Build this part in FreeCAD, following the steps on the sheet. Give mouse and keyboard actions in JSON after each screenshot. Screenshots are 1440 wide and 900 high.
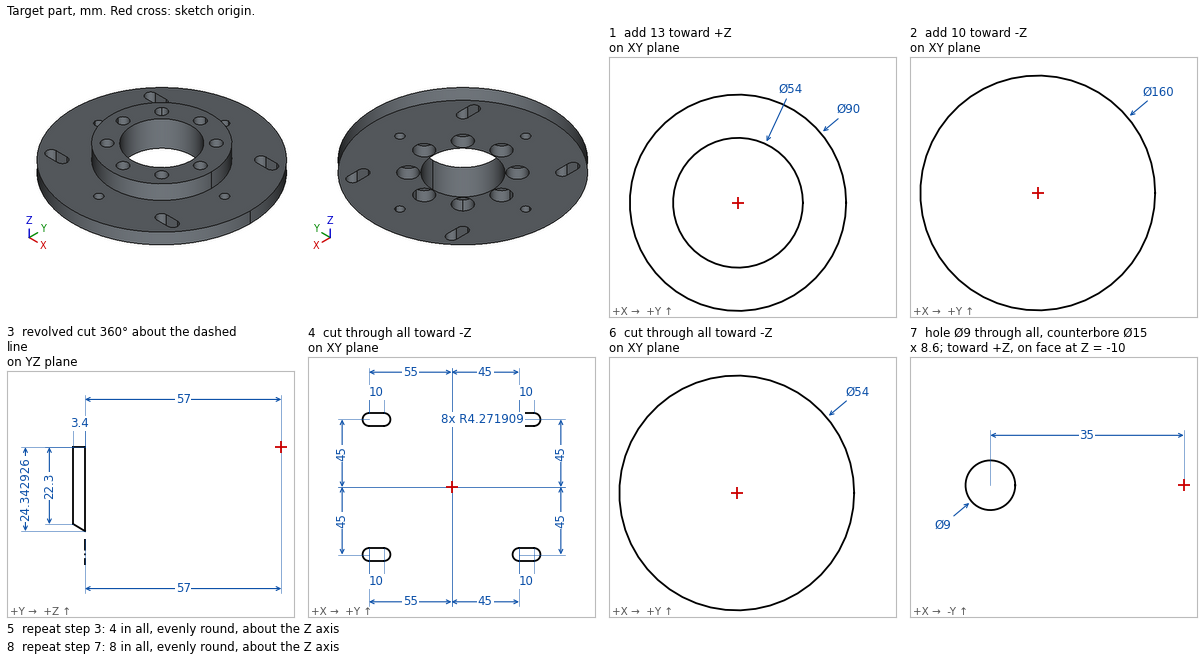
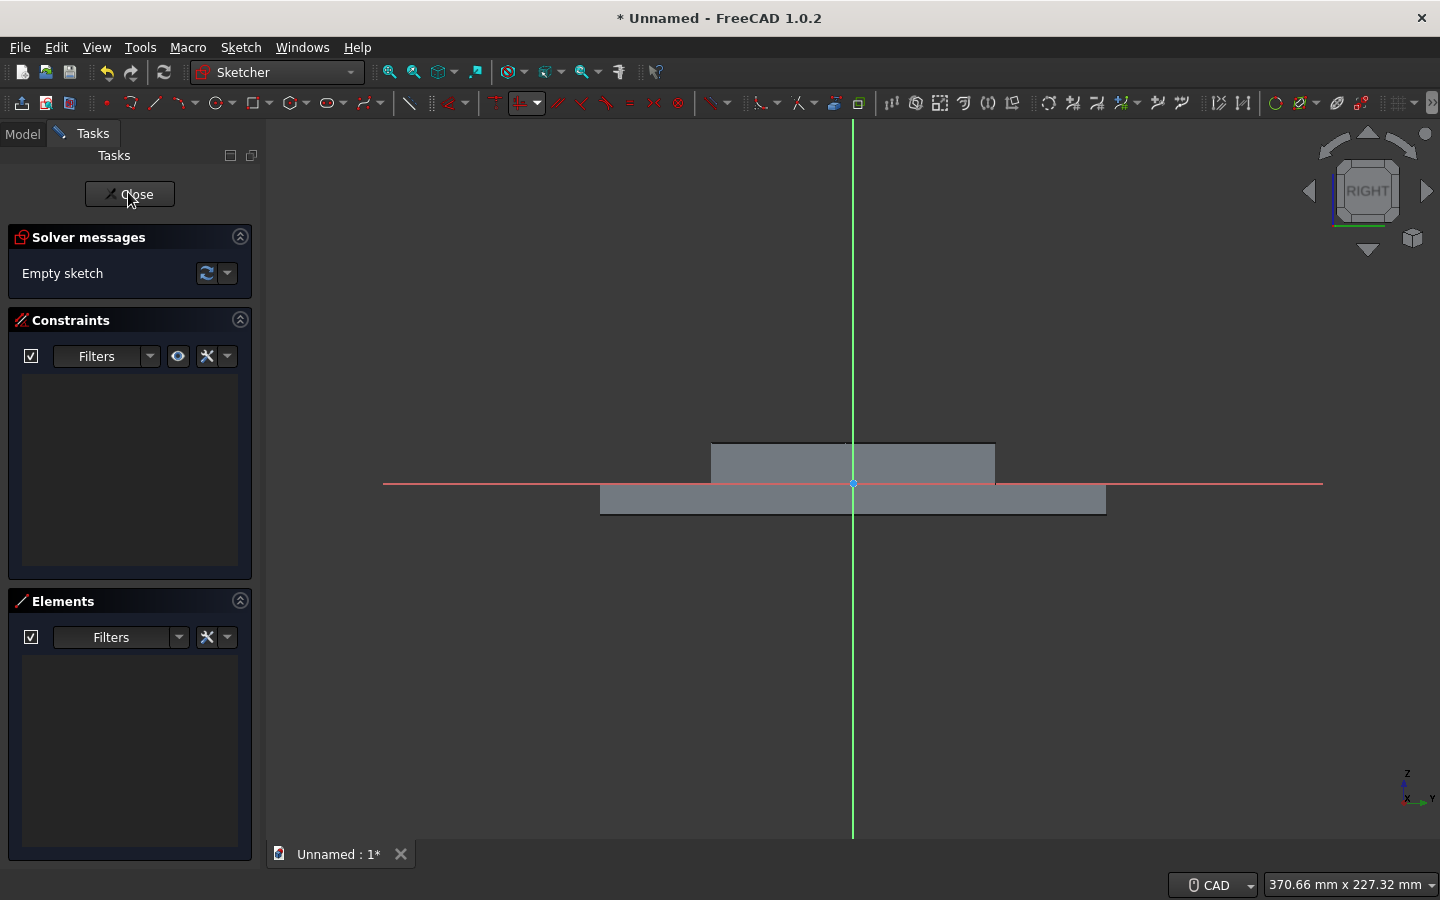
{"action": "scroll", "coordinate": [746, 563], "scroll_direction": "up", "scroll_amount": 6}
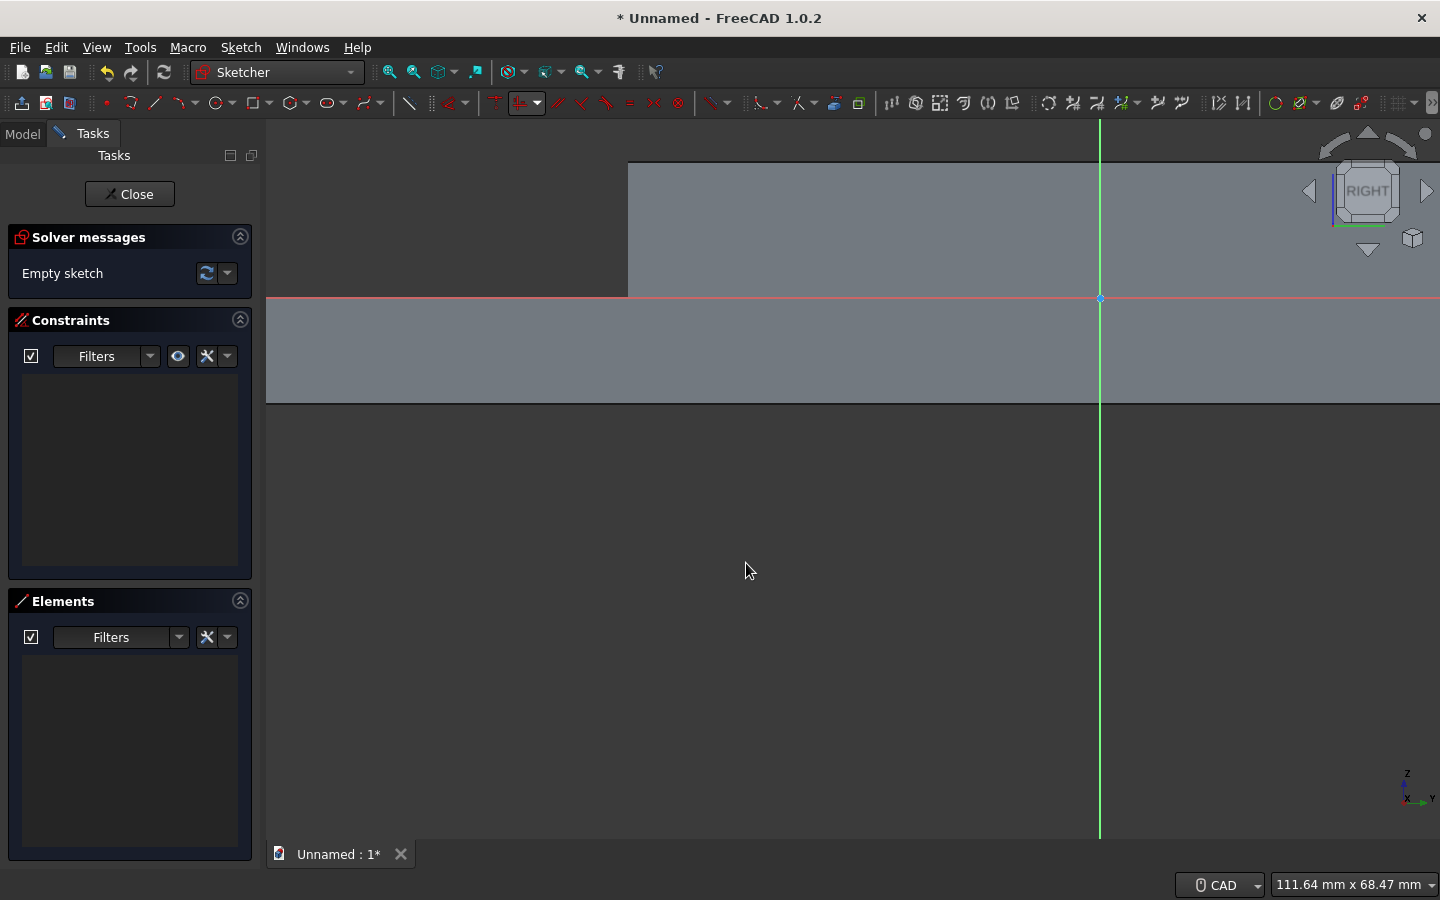
{"action": "key", "text": "g m"}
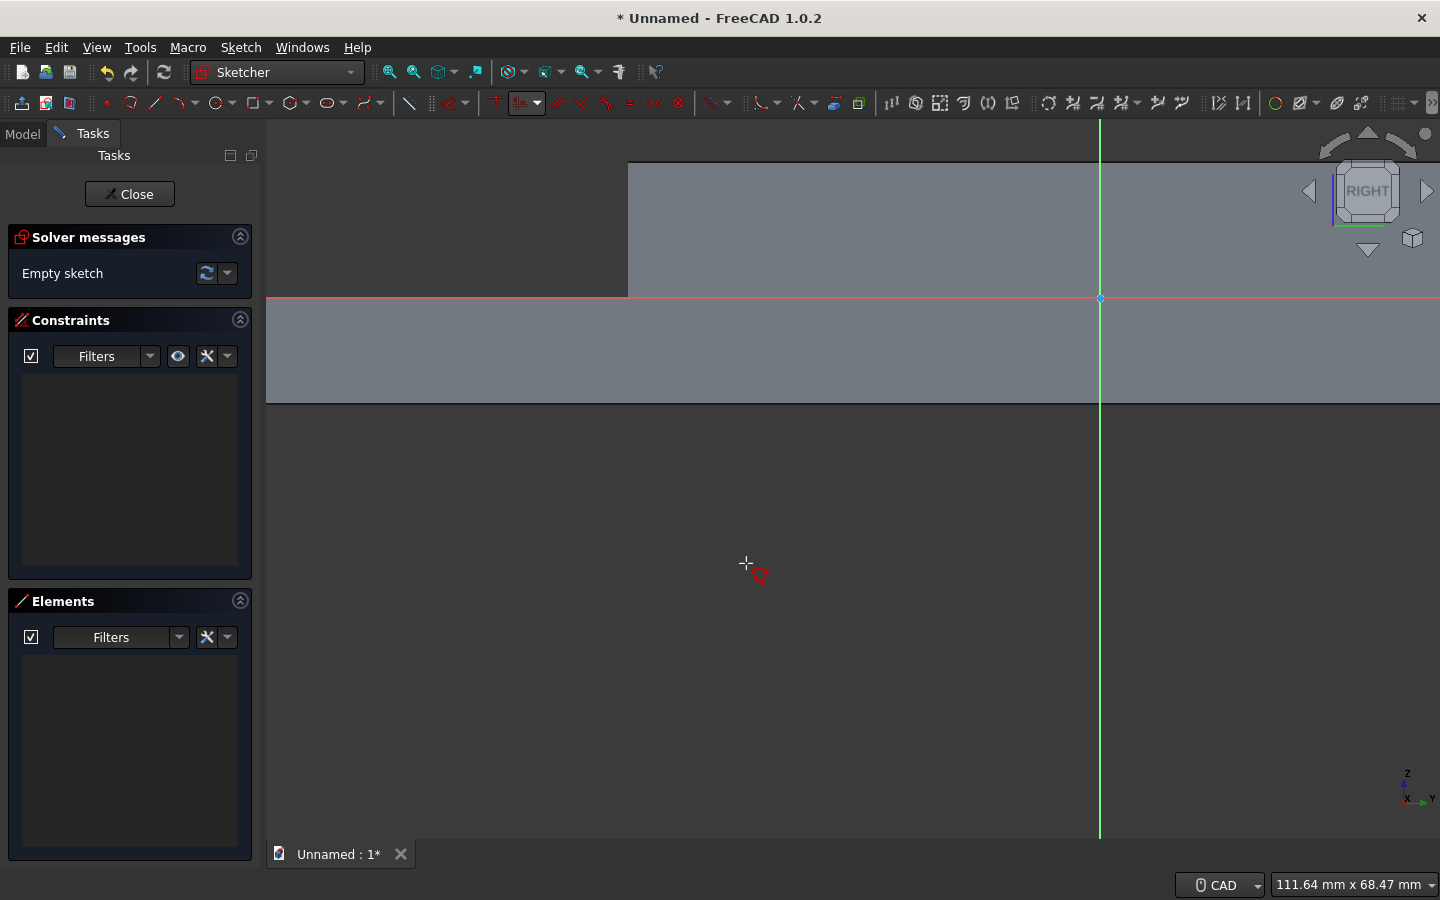
{"action": "left_click", "coordinate": [501, 298]}
{"action": "left_click", "coordinate": [465, 307]}
{"action": "left_click", "coordinate": [465, 533]}
{"action": "left_click", "coordinate": [501, 554]}
{"action": "left_click", "coordinate": [501, 298]}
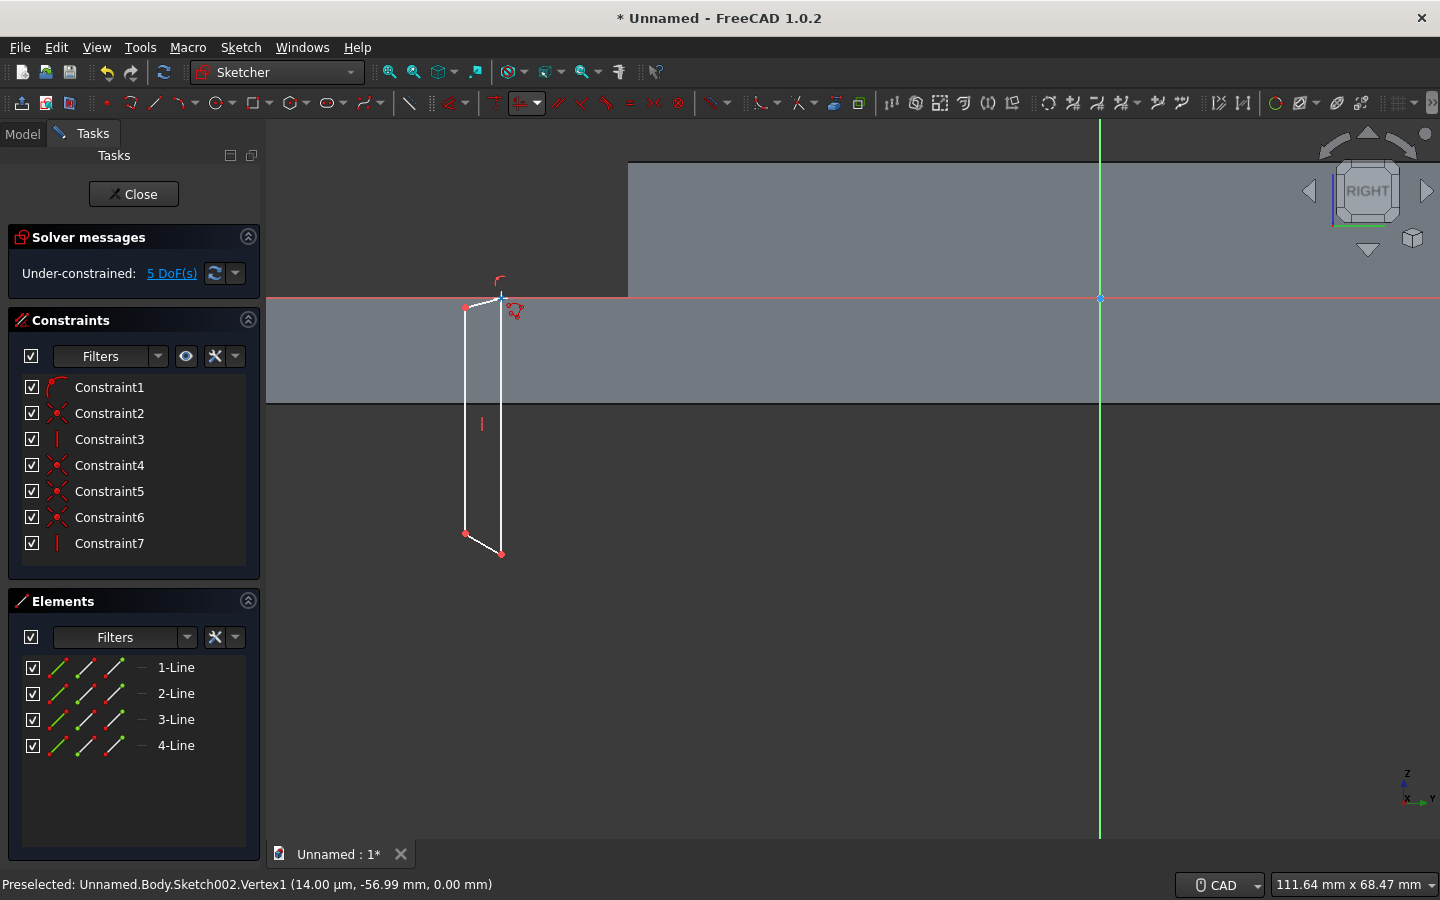
{"action": "left_click", "coordinate": [156, 104]}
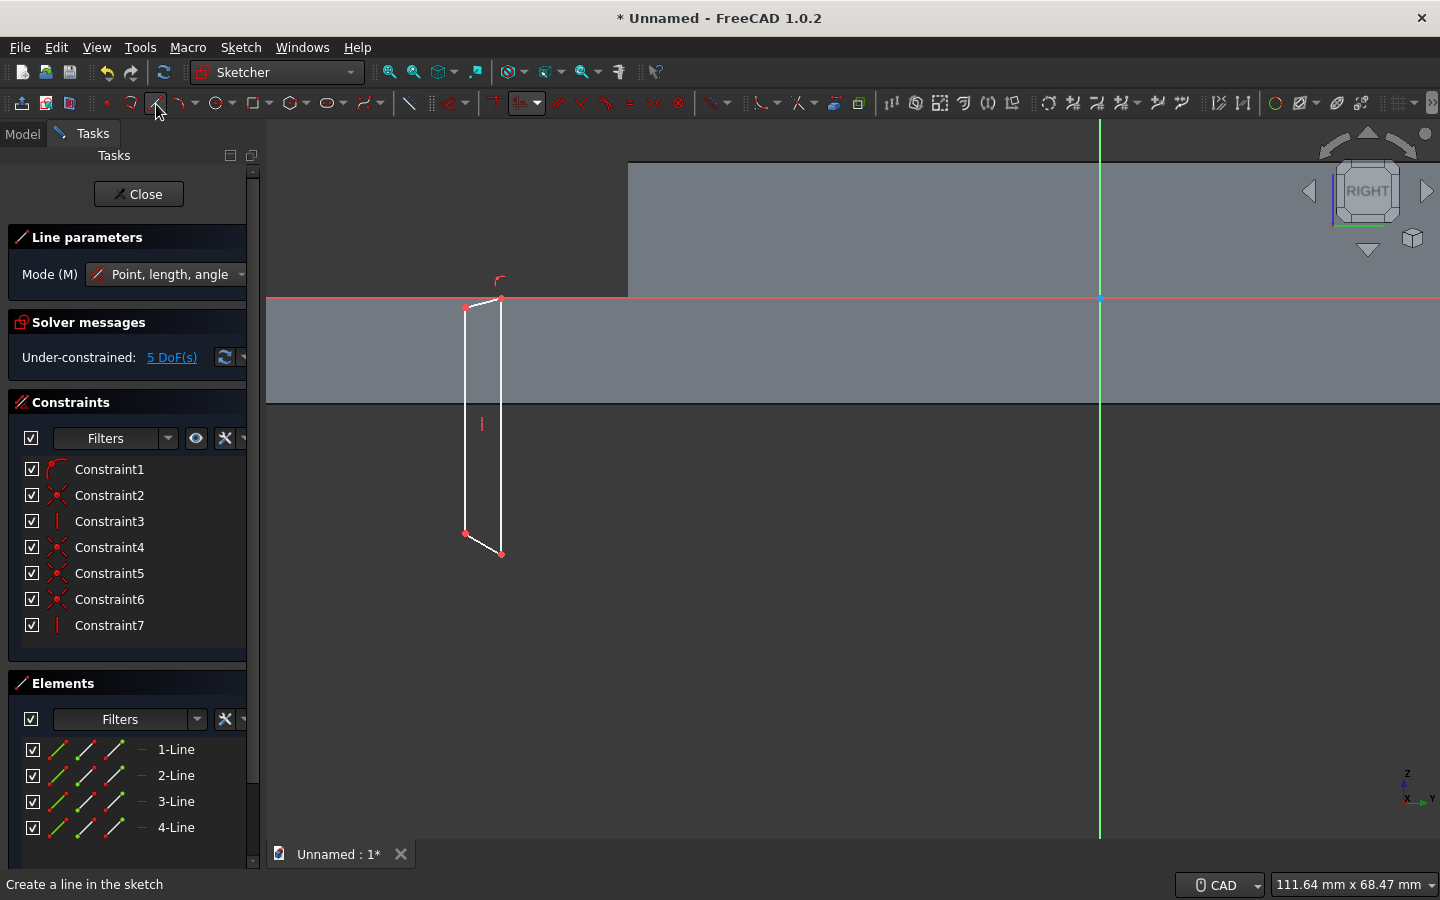
{"action": "left_click", "coordinate": [501, 580]}
{"action": "left_click", "coordinate": [501, 657]}
{"action": "key", "text": "Escape"}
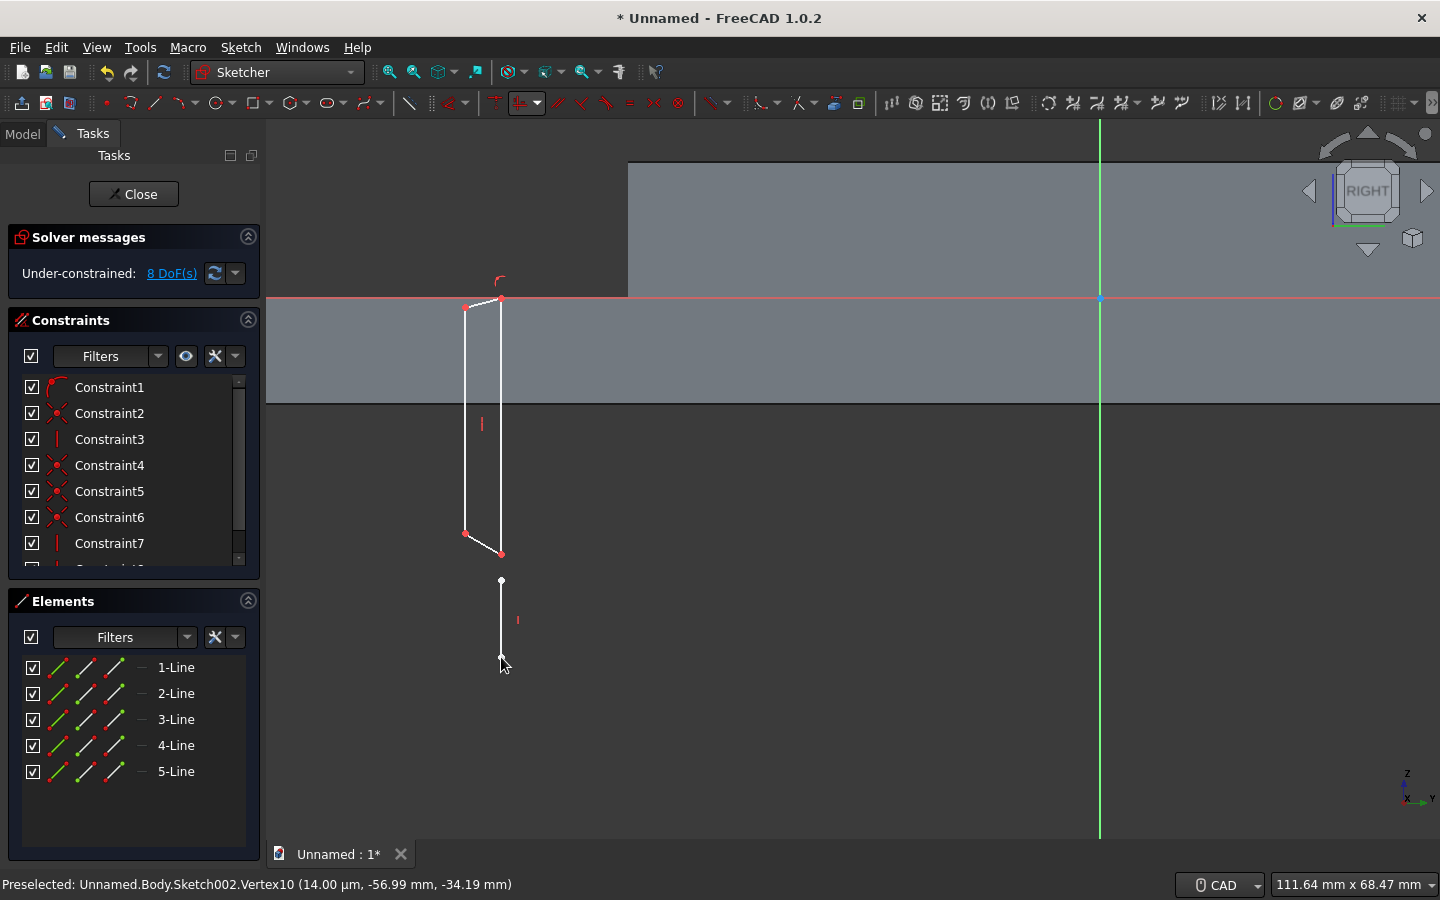
{"action": "left_click", "coordinate": [501, 604]}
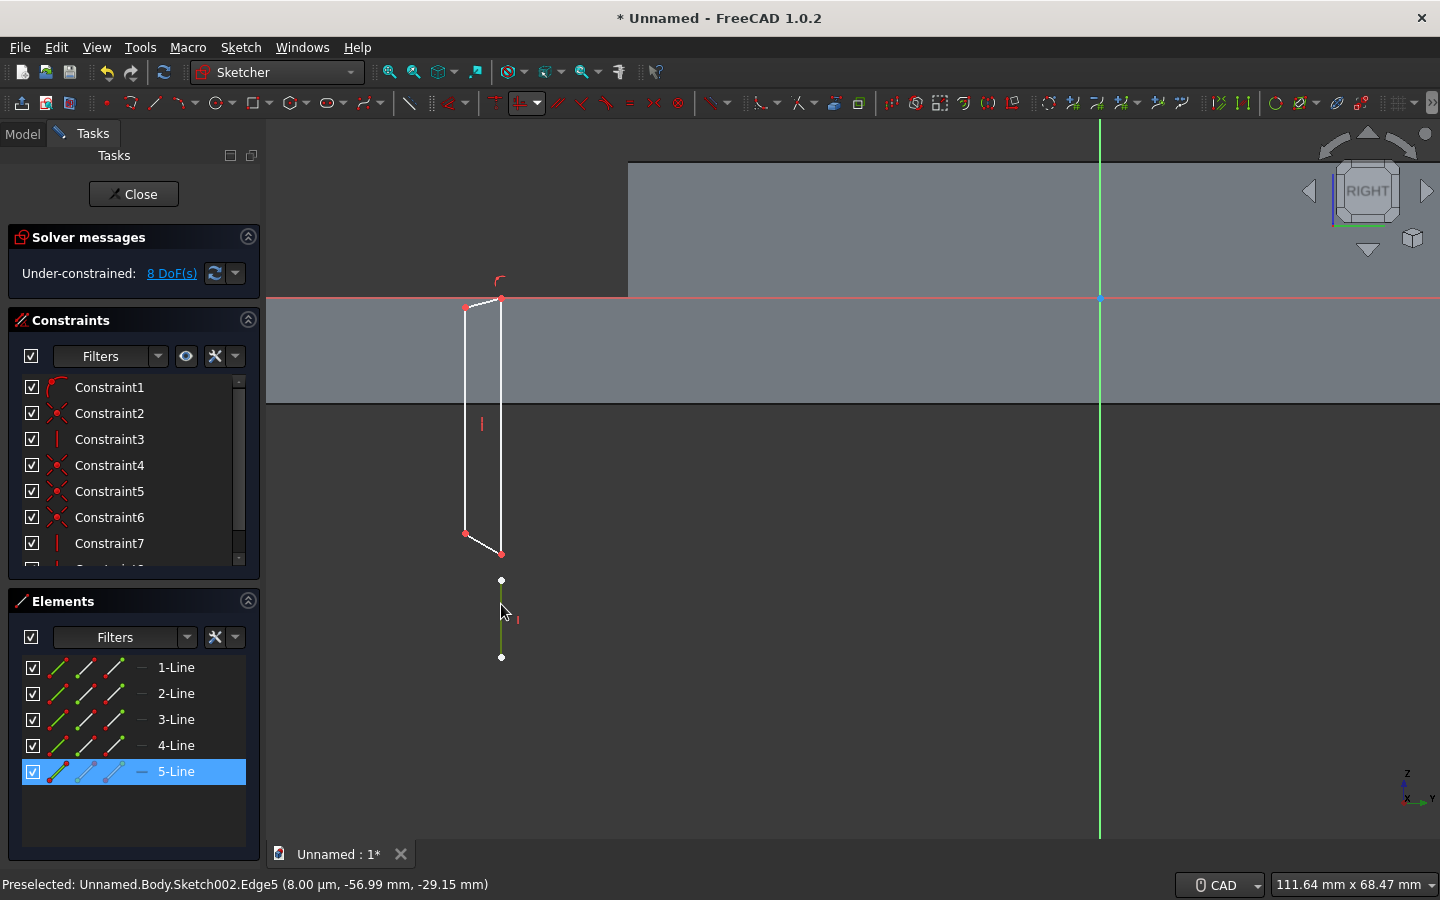
{"action": "left_click", "coordinate": [410, 104]}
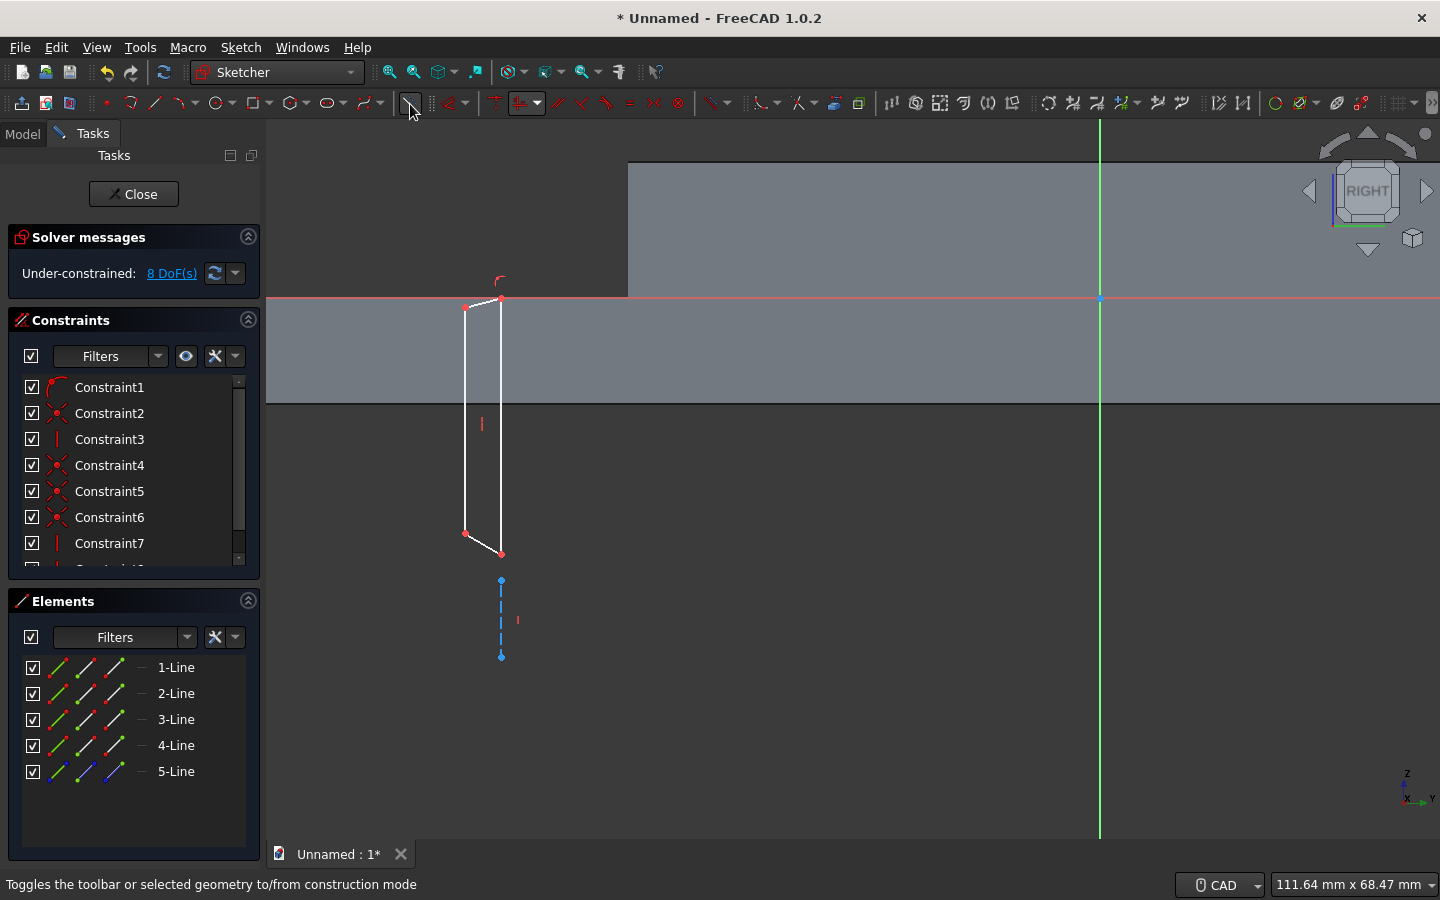
{"action": "scroll", "coordinate": [490, 301], "scroll_direction": "up", "scroll_amount": 2}